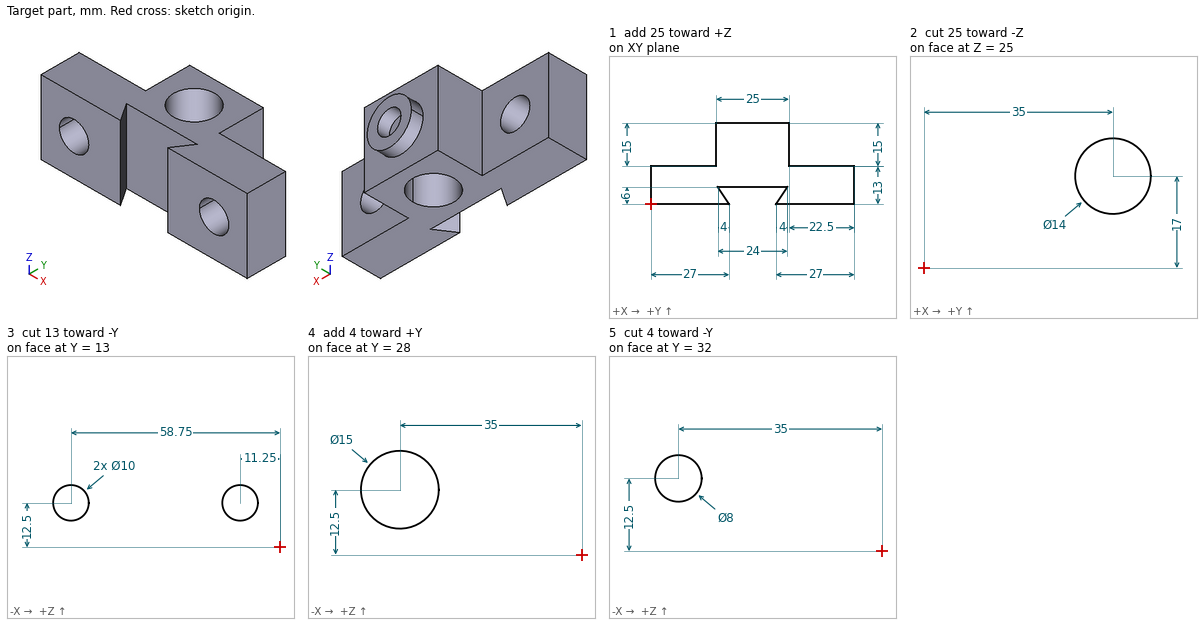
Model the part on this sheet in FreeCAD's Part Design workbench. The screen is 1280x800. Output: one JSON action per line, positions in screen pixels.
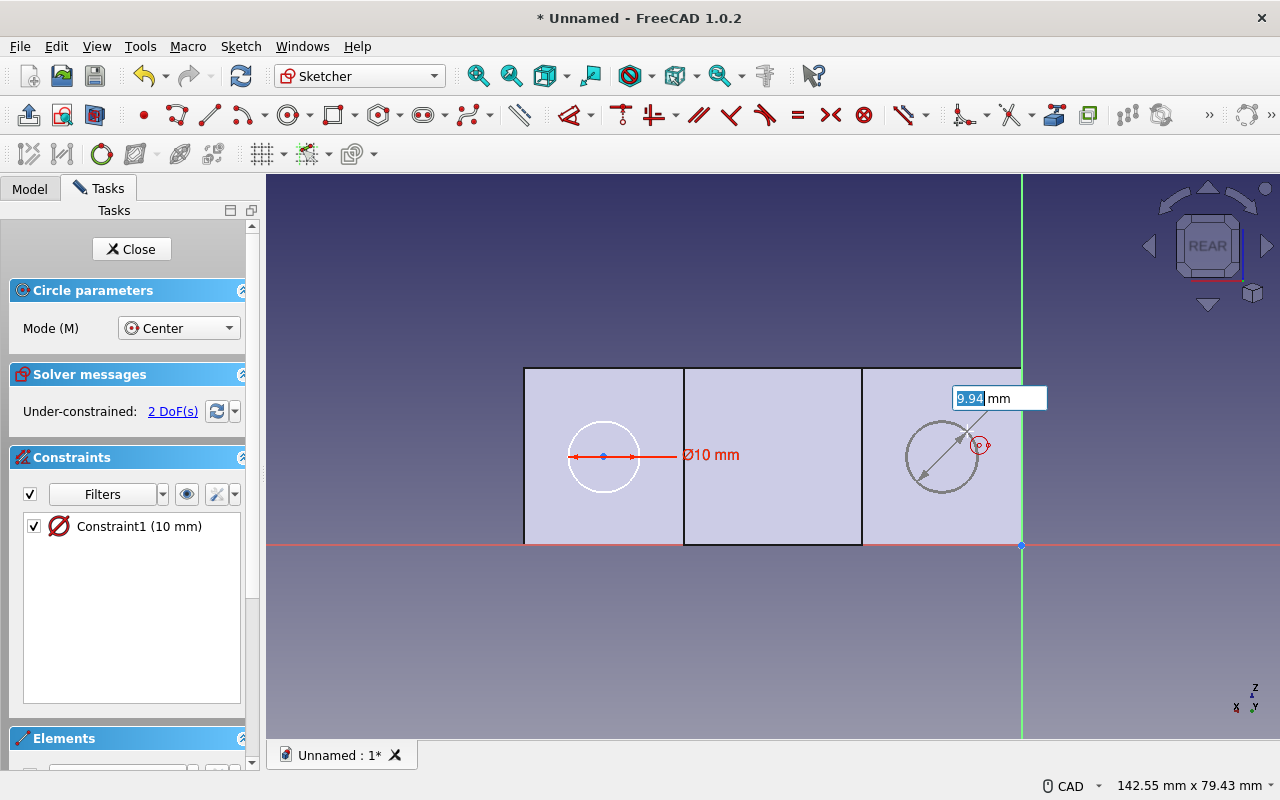
{"action": "type", "text": "10"}
{"action": "key", "text": "Return"}
{"action": "key", "text": "Escape"}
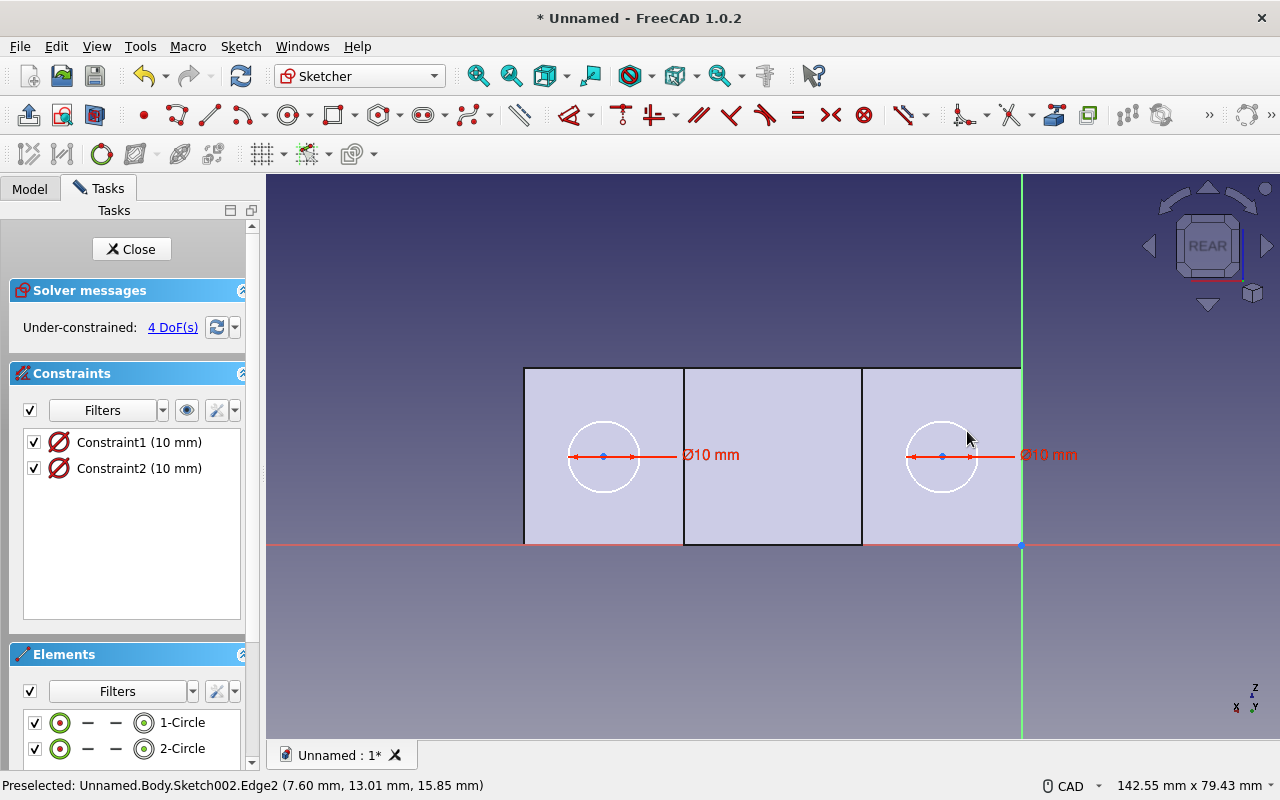
{"action": "left_click", "coordinate": [604, 457]}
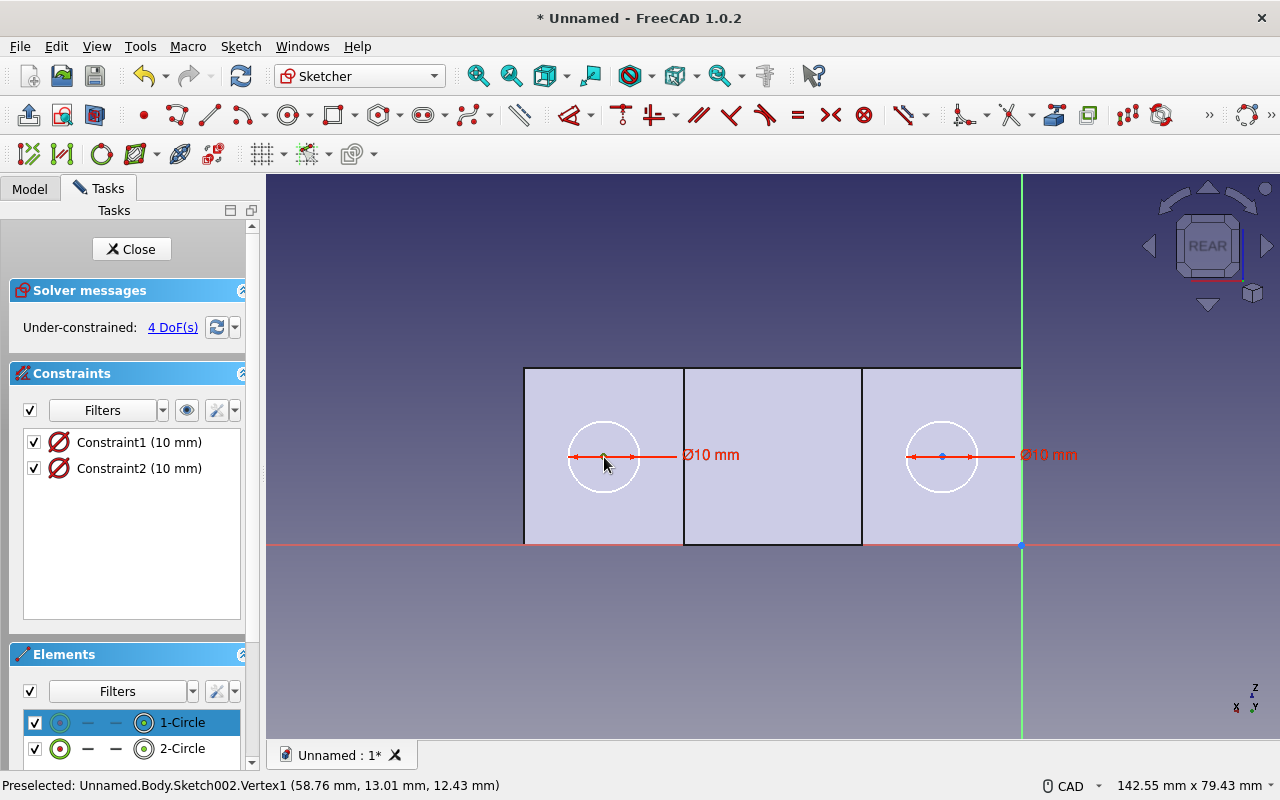
{"action": "left_click", "coordinate": [942, 457]}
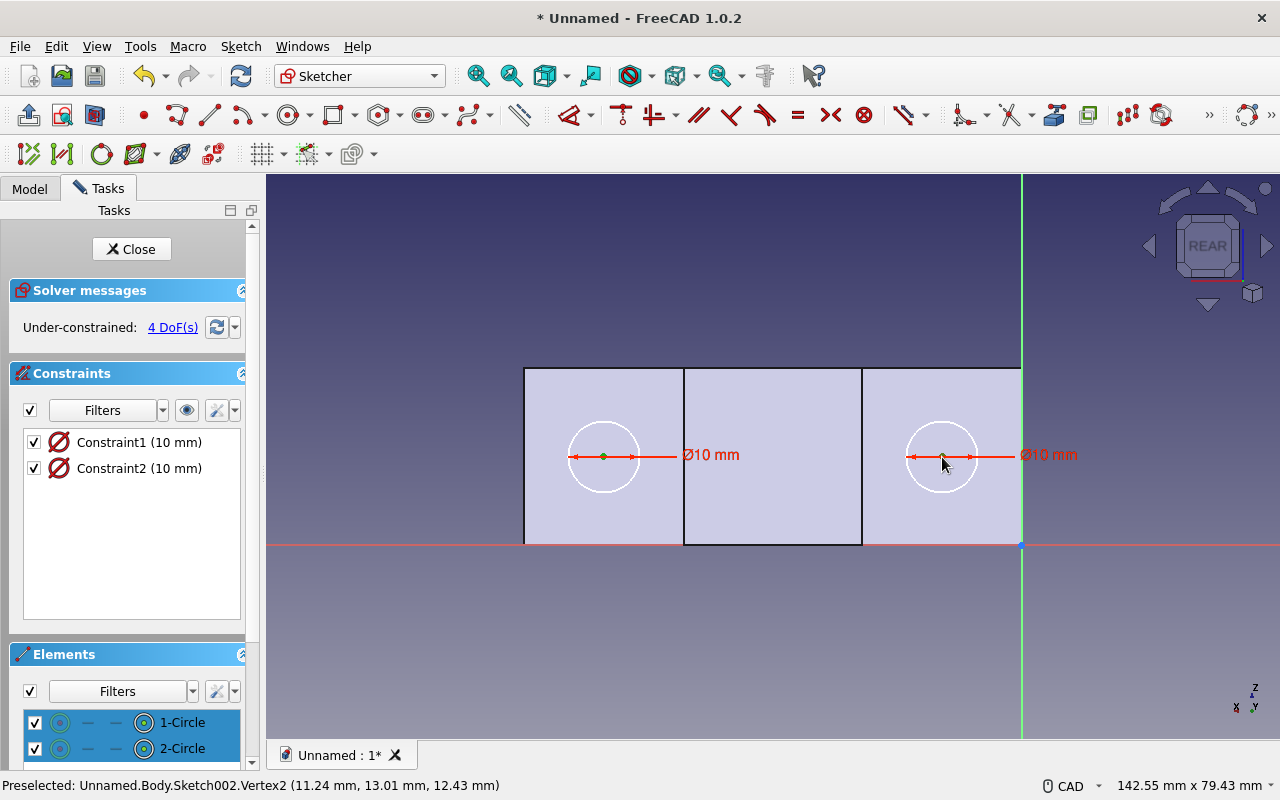
{"action": "key", "text": "h"}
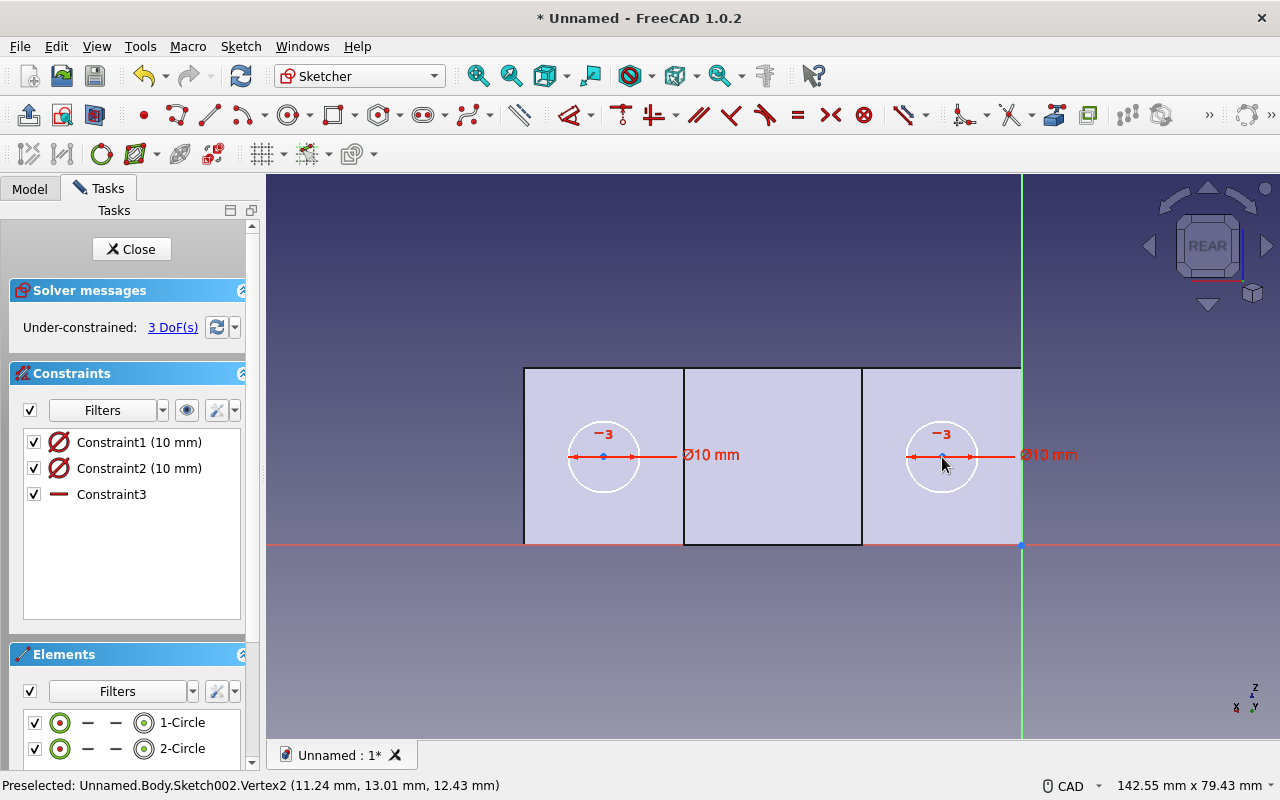
{"action": "left_click", "coordinate": [568, 116]}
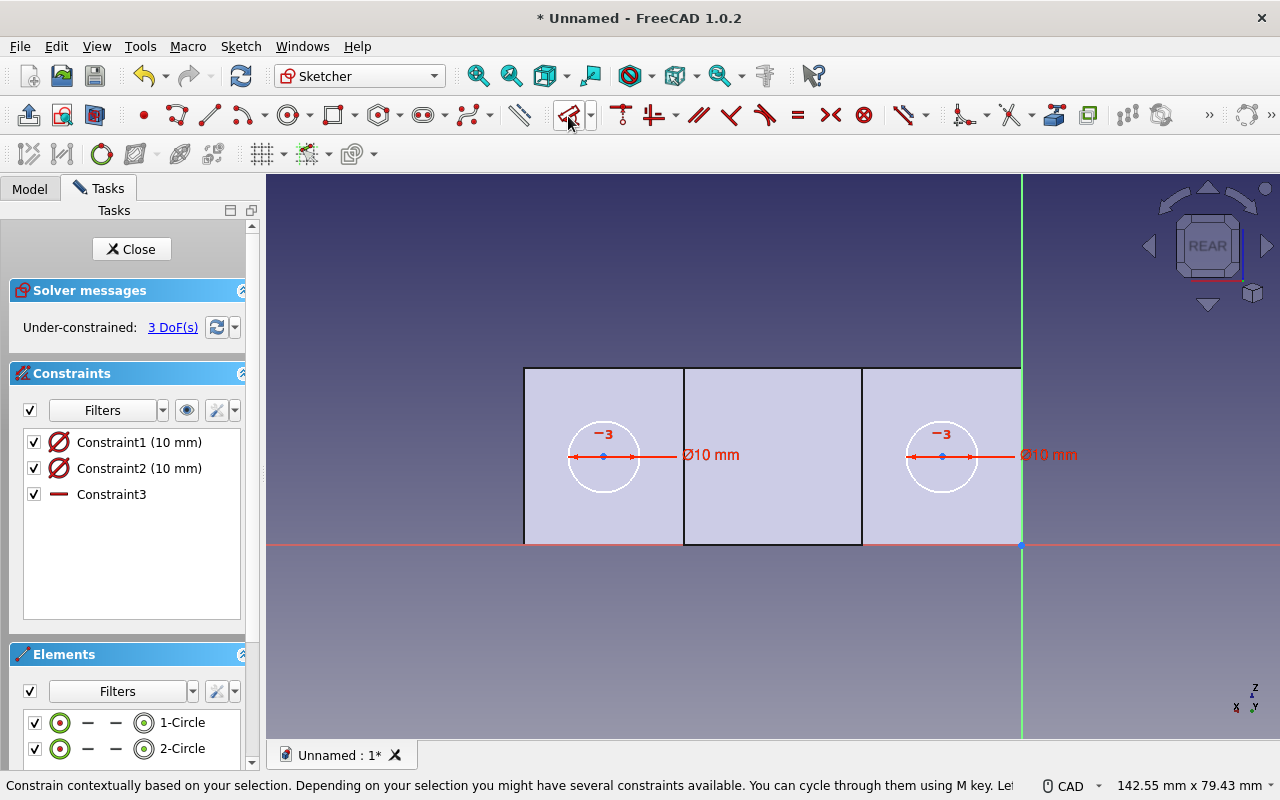
{"action": "left_click", "coordinate": [604, 457]}
{"action": "left_click", "coordinate": [1056, 501]}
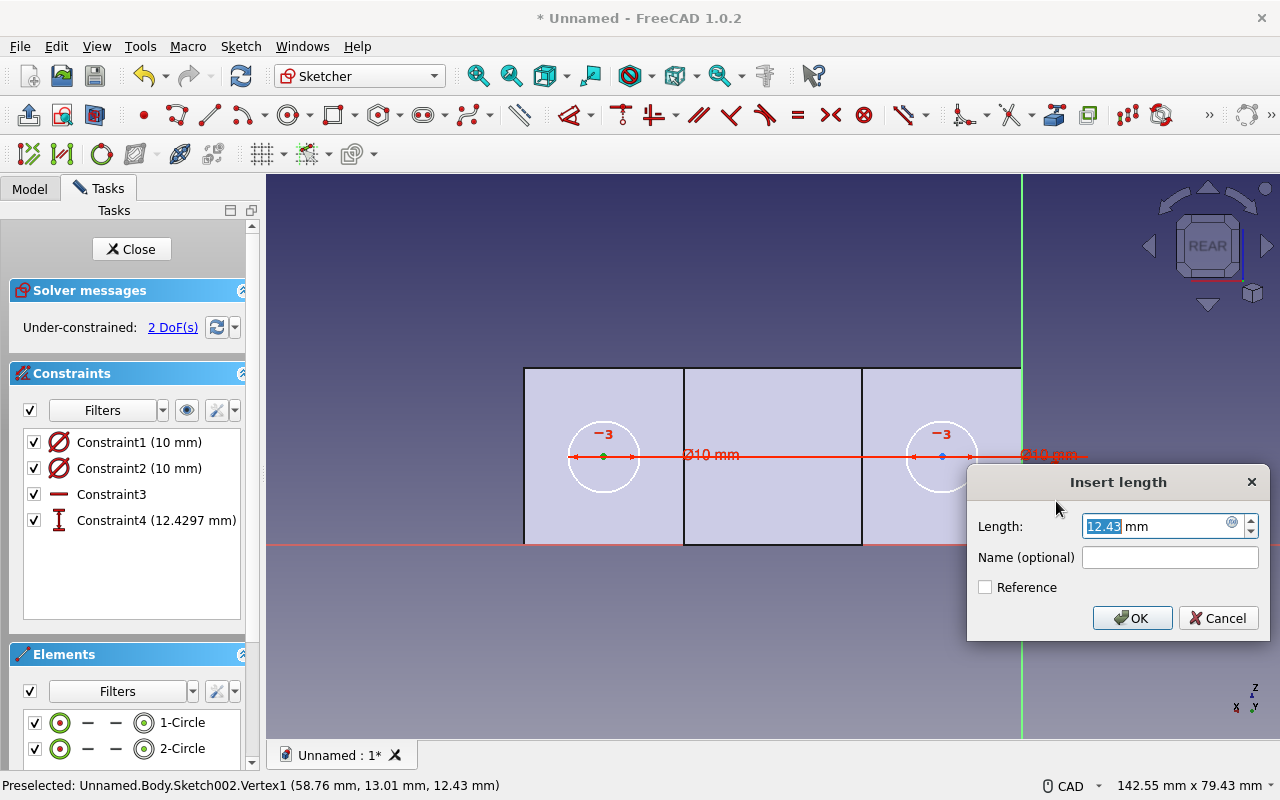
{"action": "type", "text": "12.5"}
{"action": "key", "text": "Return"}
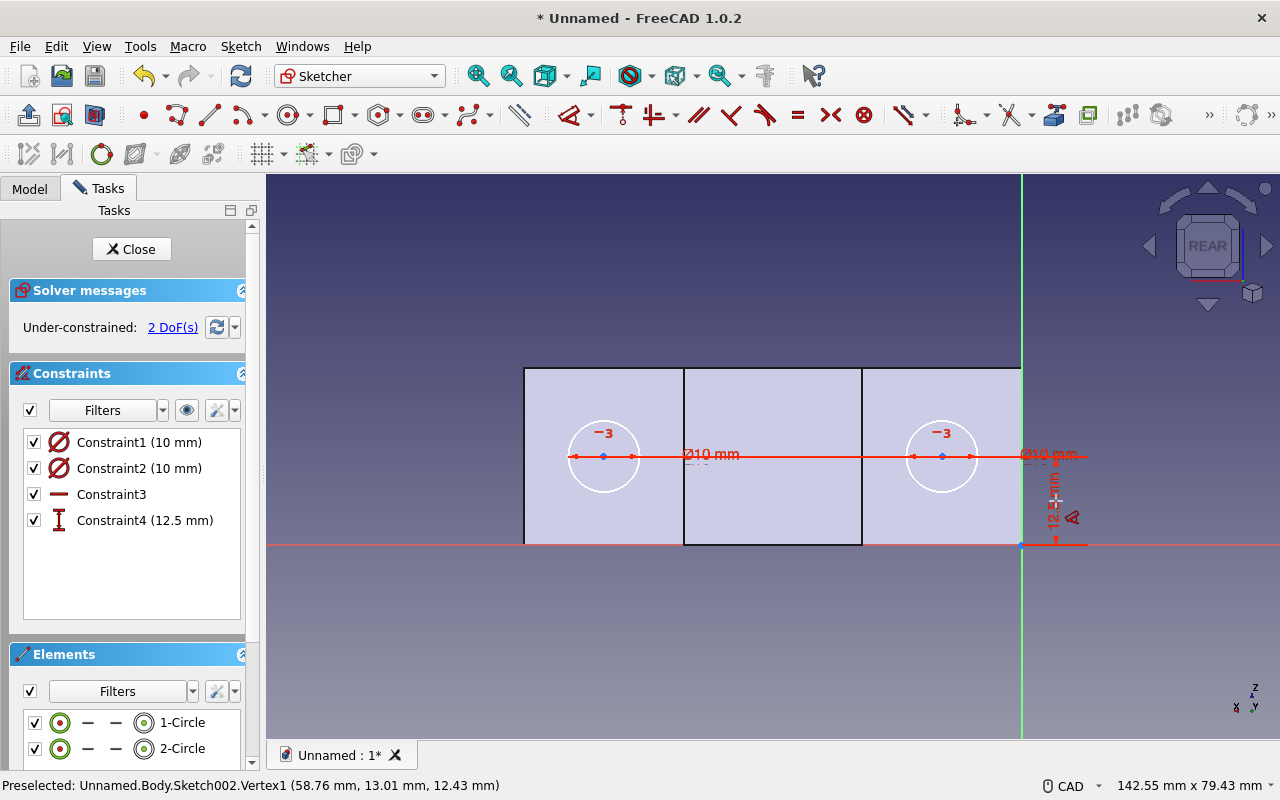
{"action": "left_click", "coordinate": [604, 456]}
{"action": "left_click", "coordinate": [813, 579]}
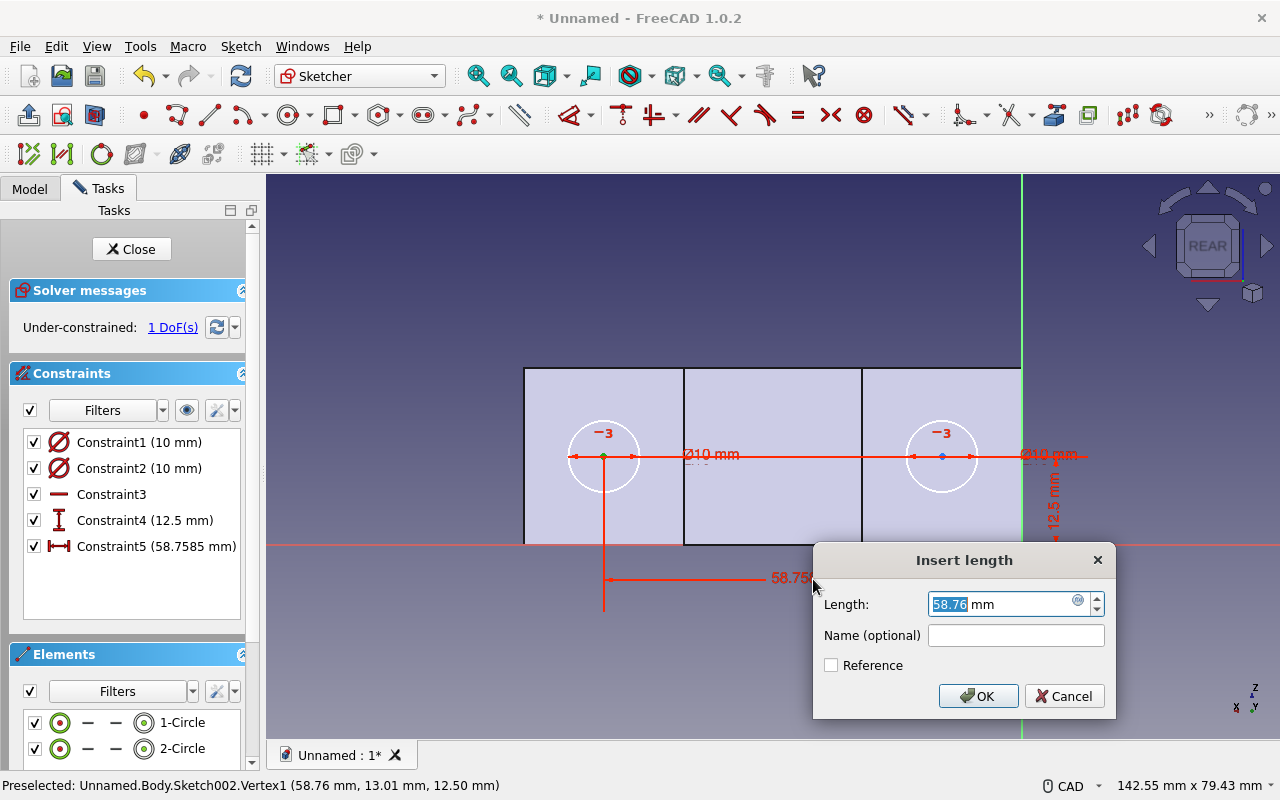
{"action": "type", "text": "58.75"}
{"action": "key", "text": "Return"}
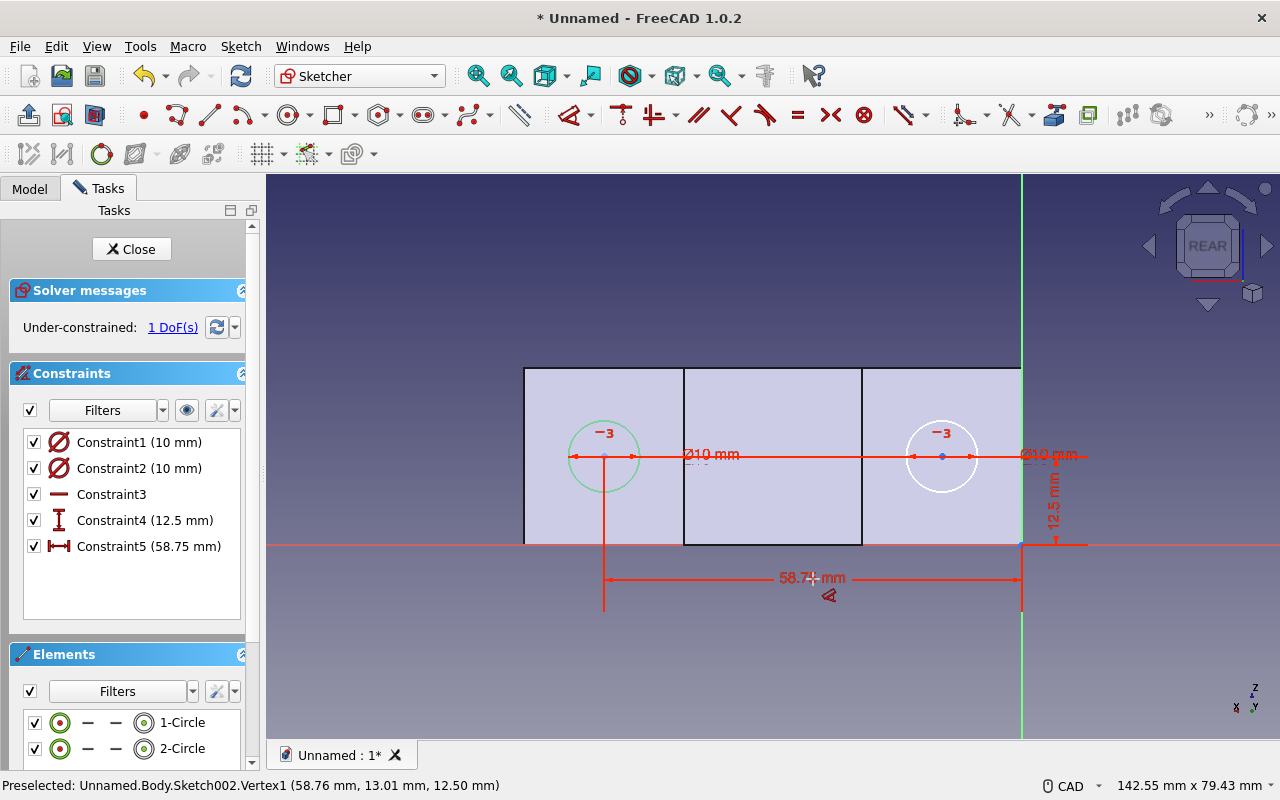
{"action": "left_click", "coordinate": [942, 456]}
{"action": "left_click", "coordinate": [982, 579]}